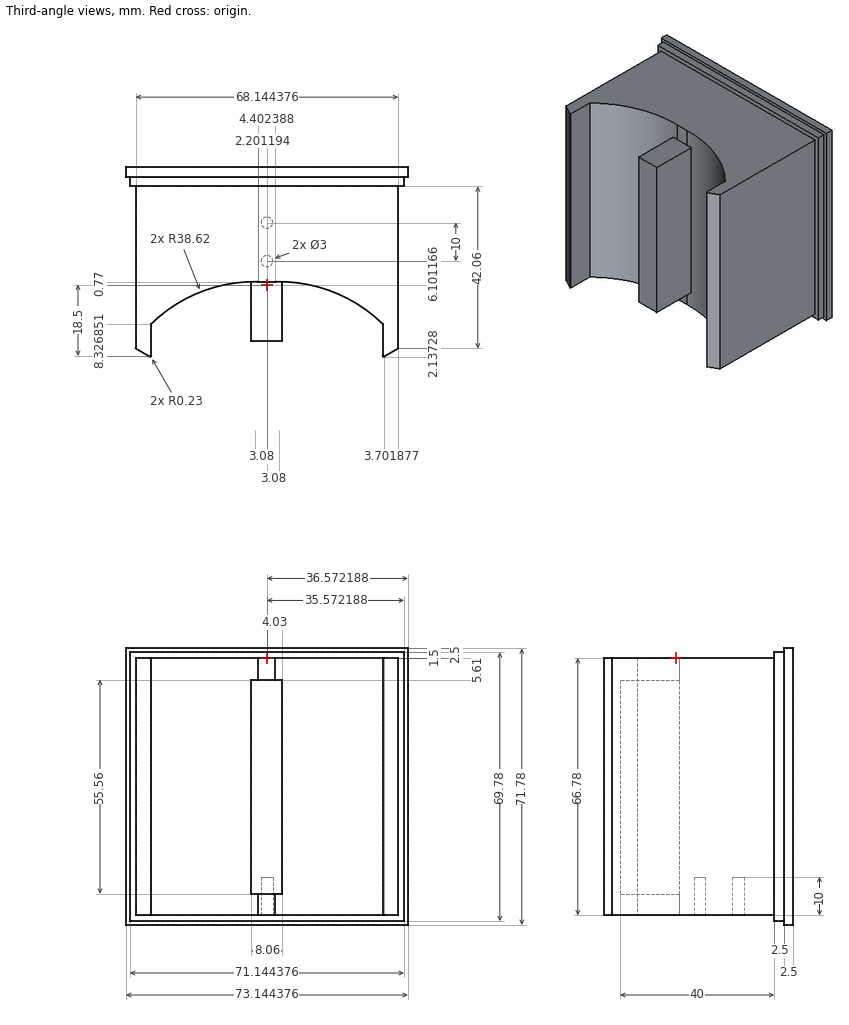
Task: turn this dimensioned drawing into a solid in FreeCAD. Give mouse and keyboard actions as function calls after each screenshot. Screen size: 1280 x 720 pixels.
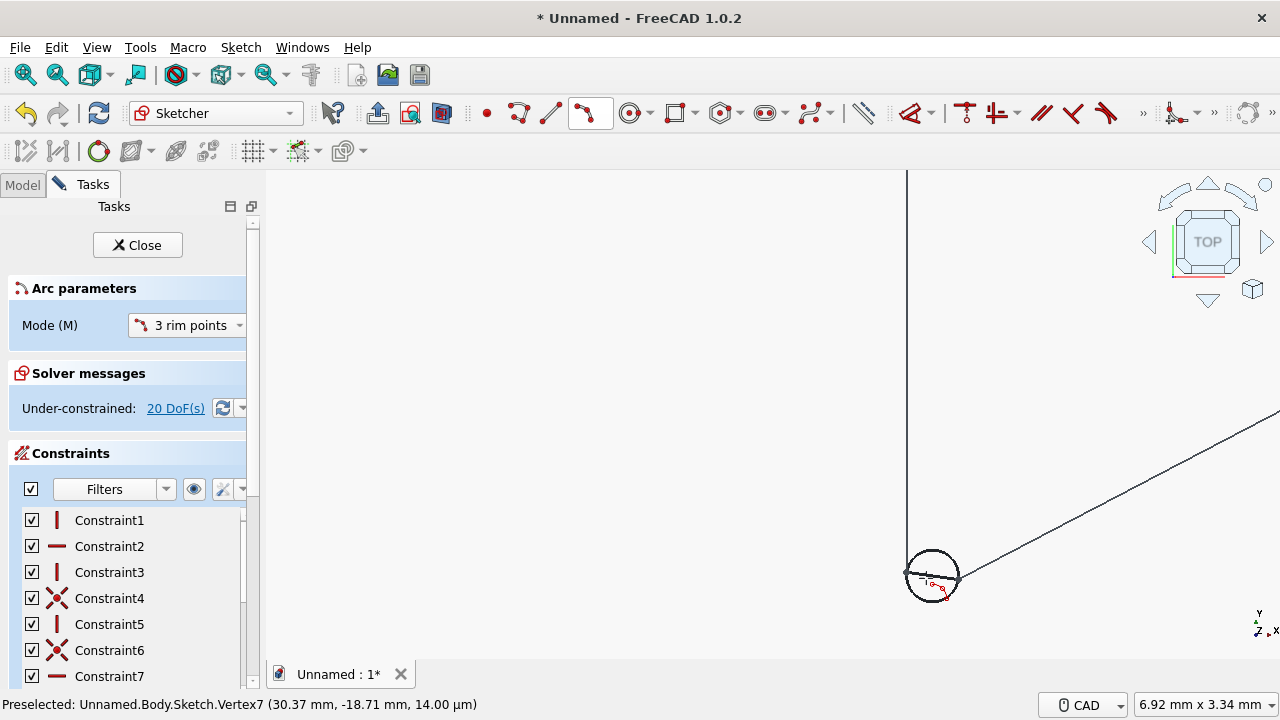
click(925, 577)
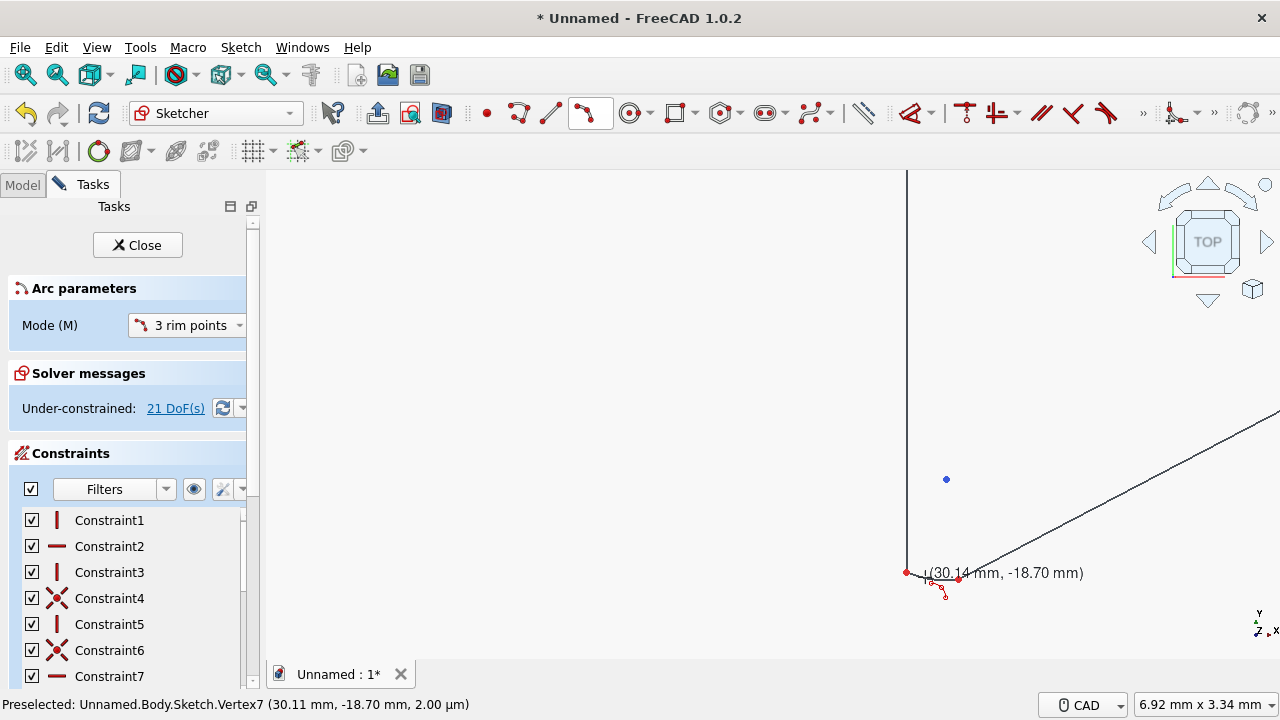
scroll(924, 576, down, 15)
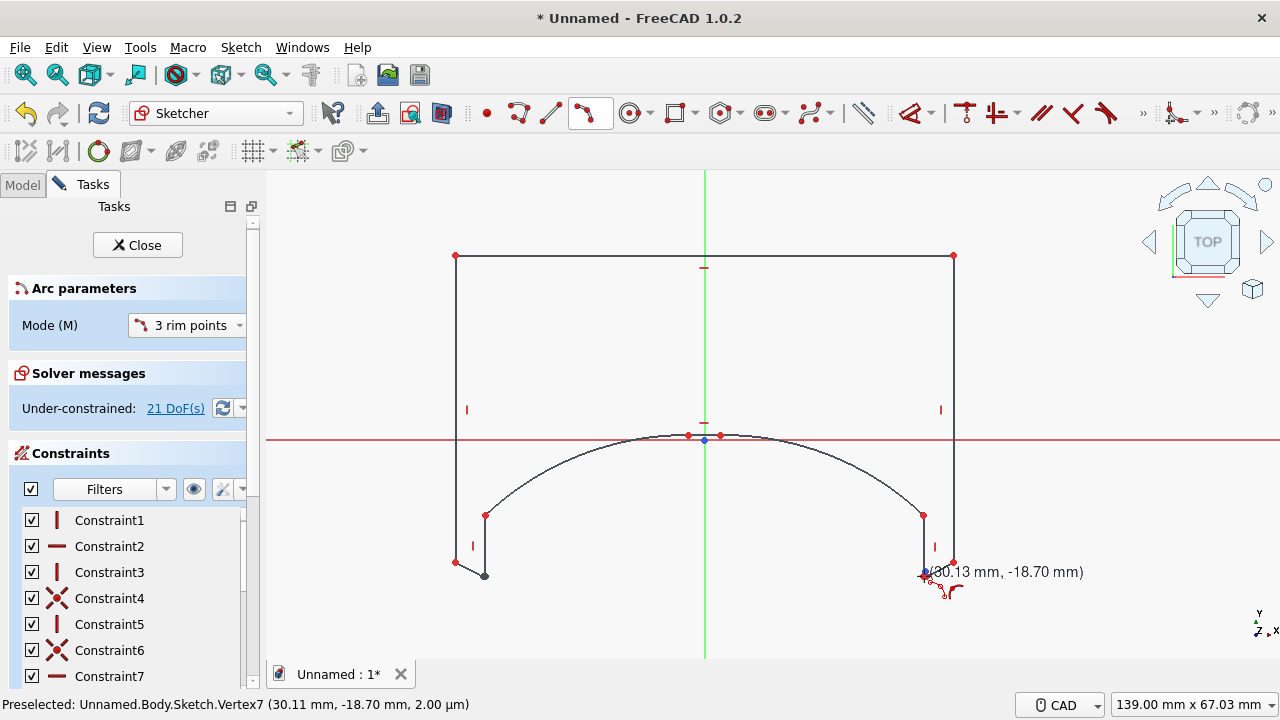
scroll(483, 577, up, 9)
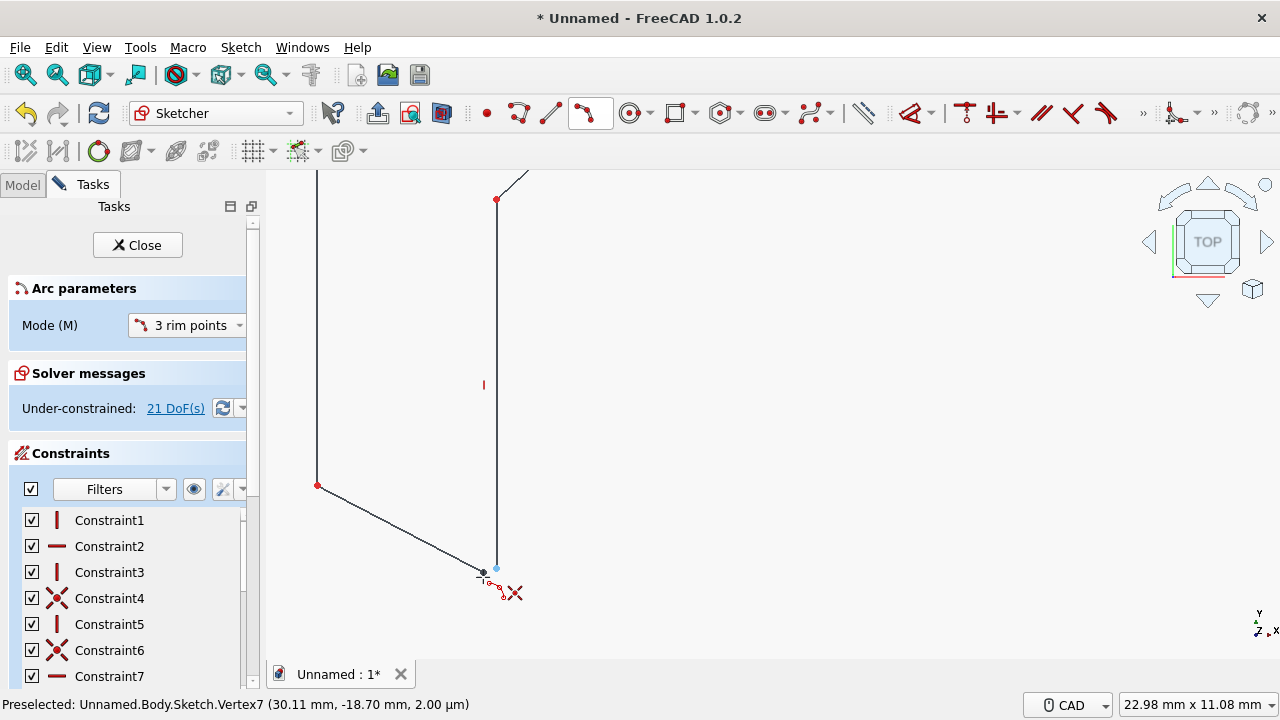
click(484, 573)
click(497, 569)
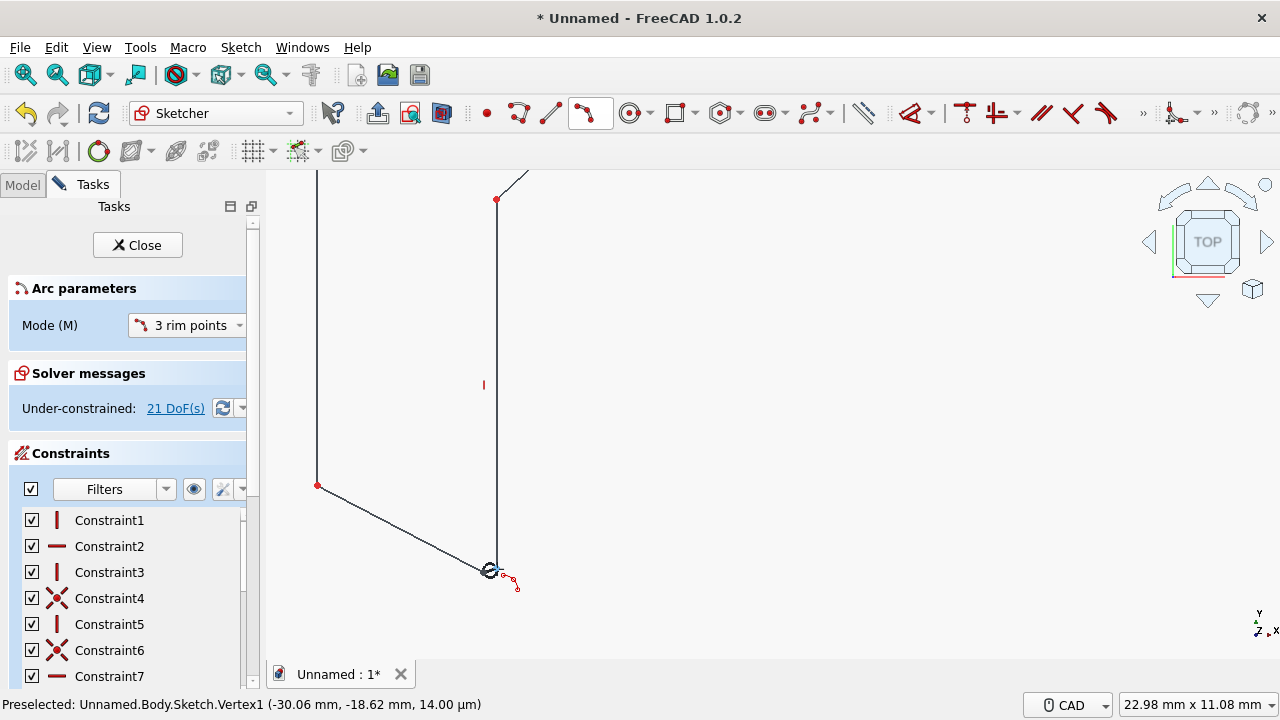
scroll(494, 572, up, 6)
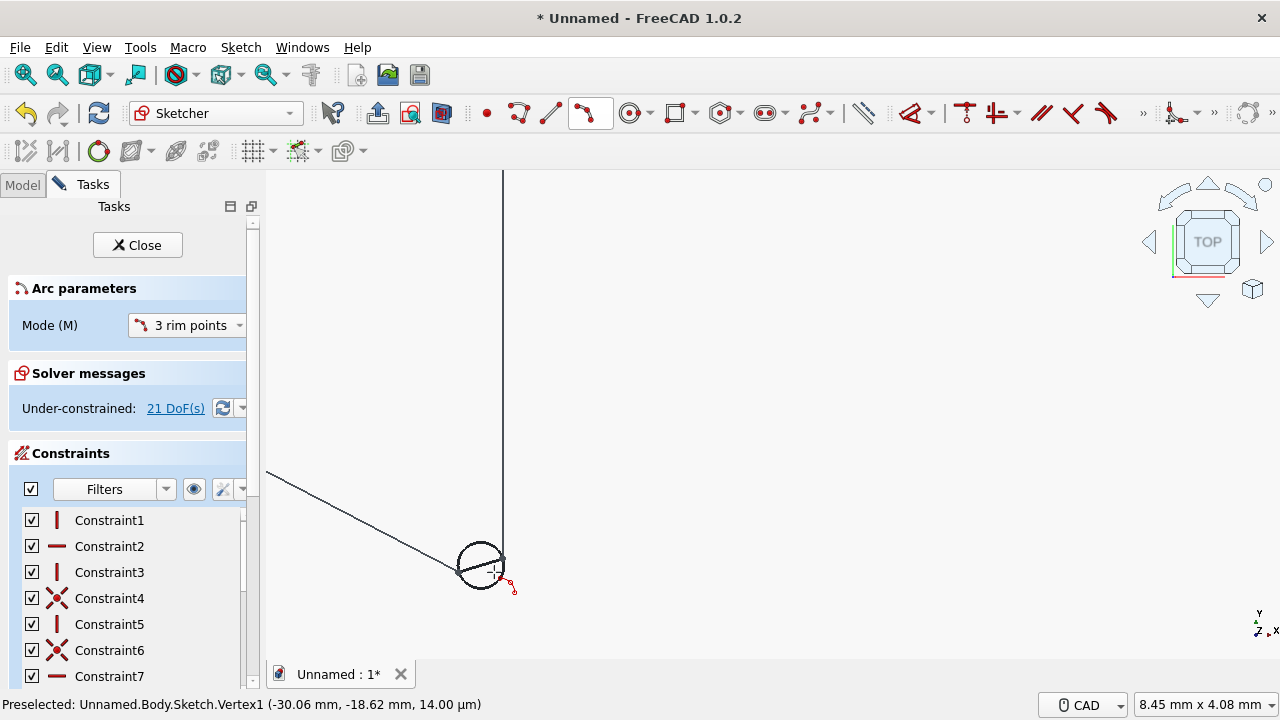
click(492, 570)
key(Escape)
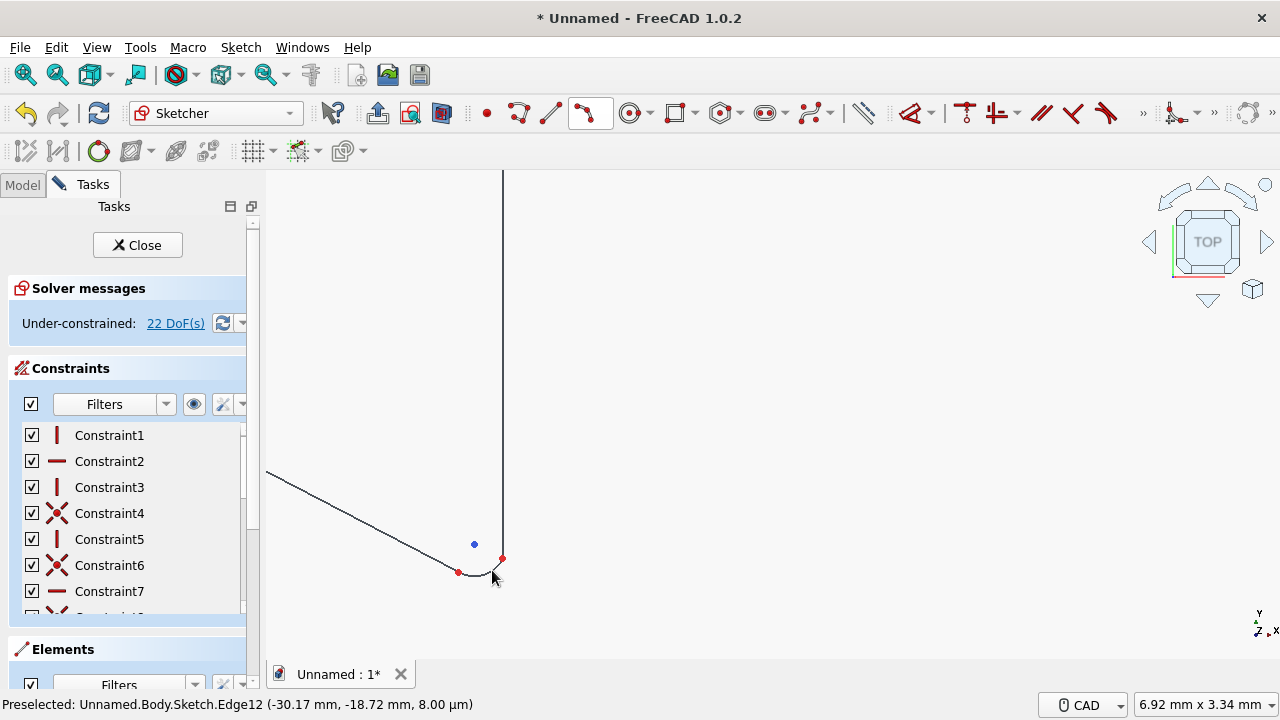
scroll(484, 576, down, 15)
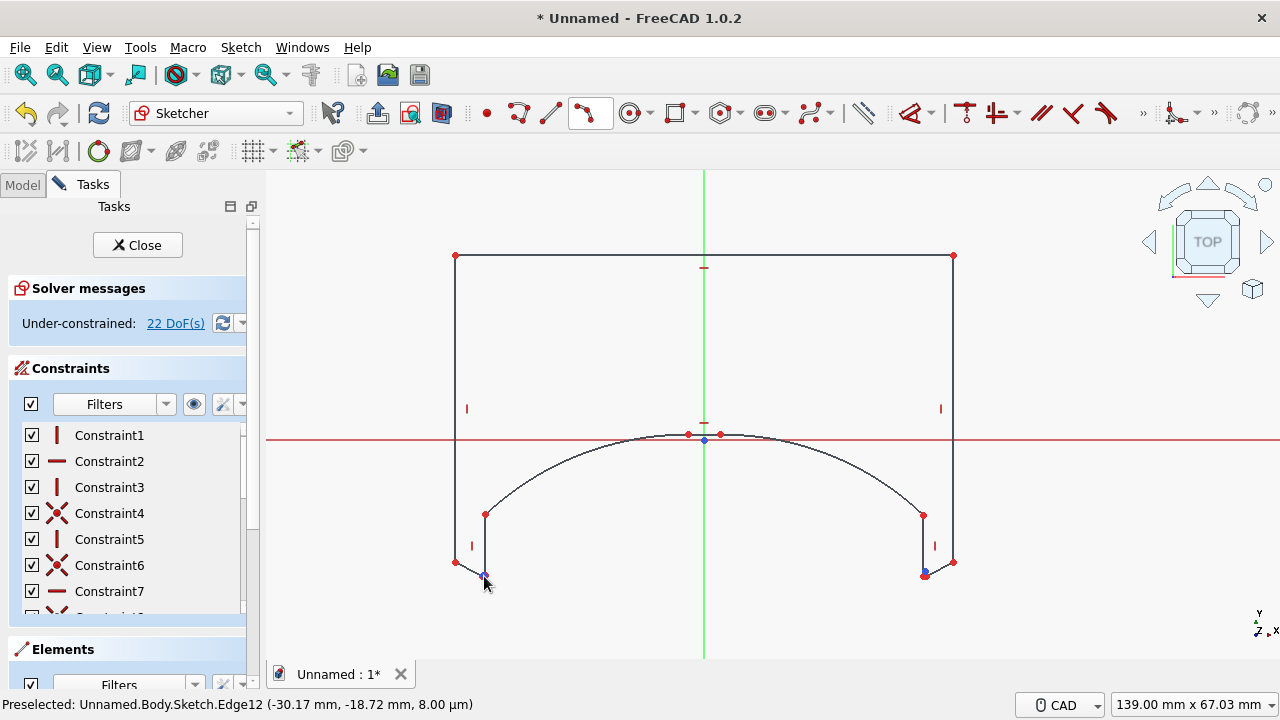
click(485, 564)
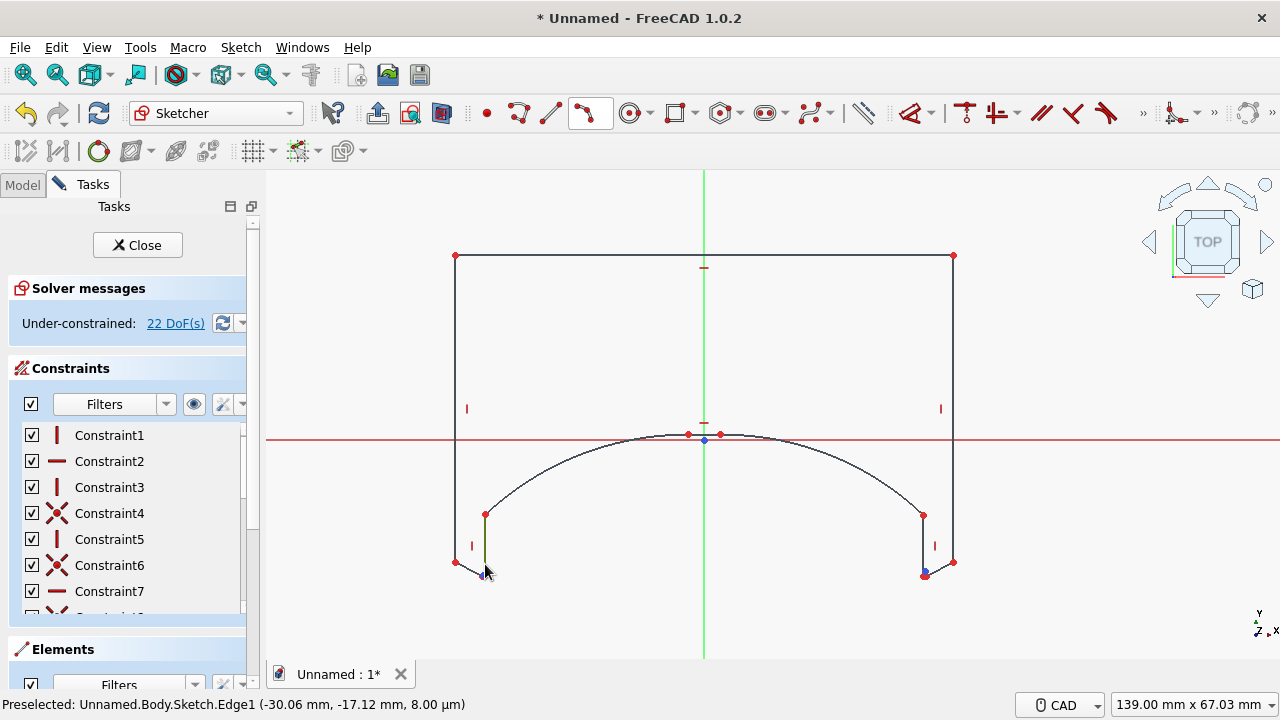
scroll(484, 577, up, 13)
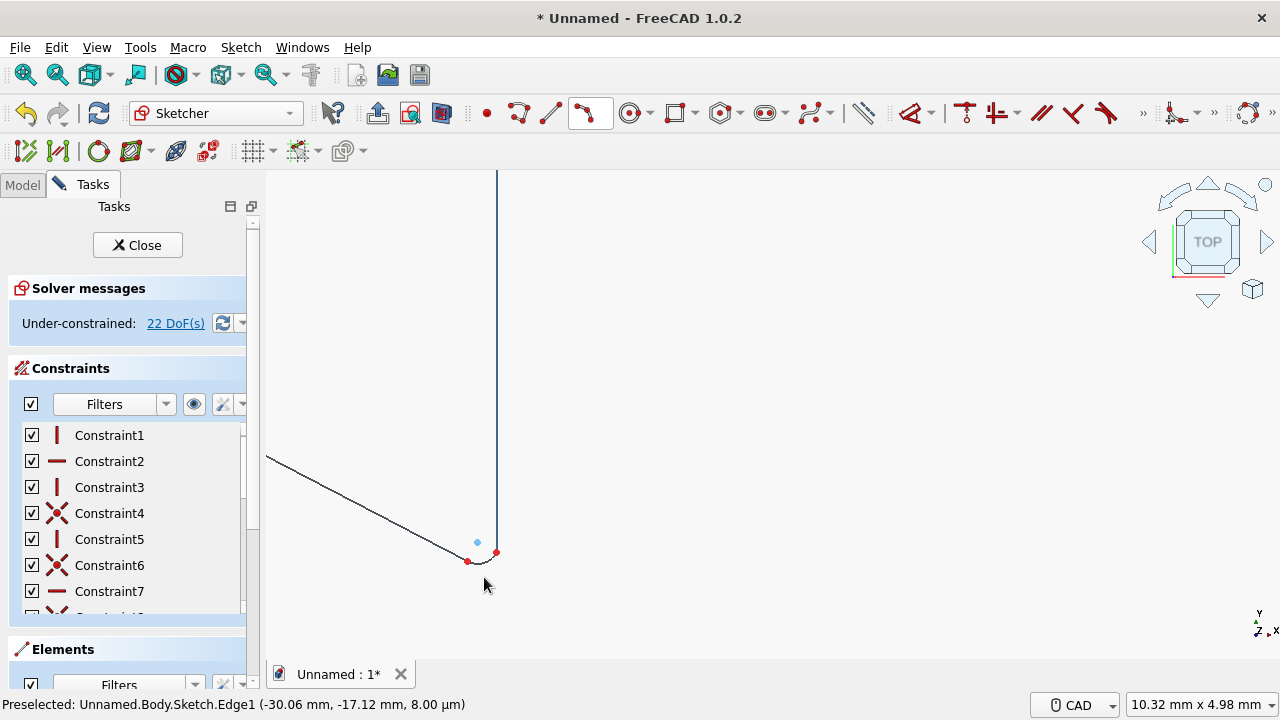
click(484, 563)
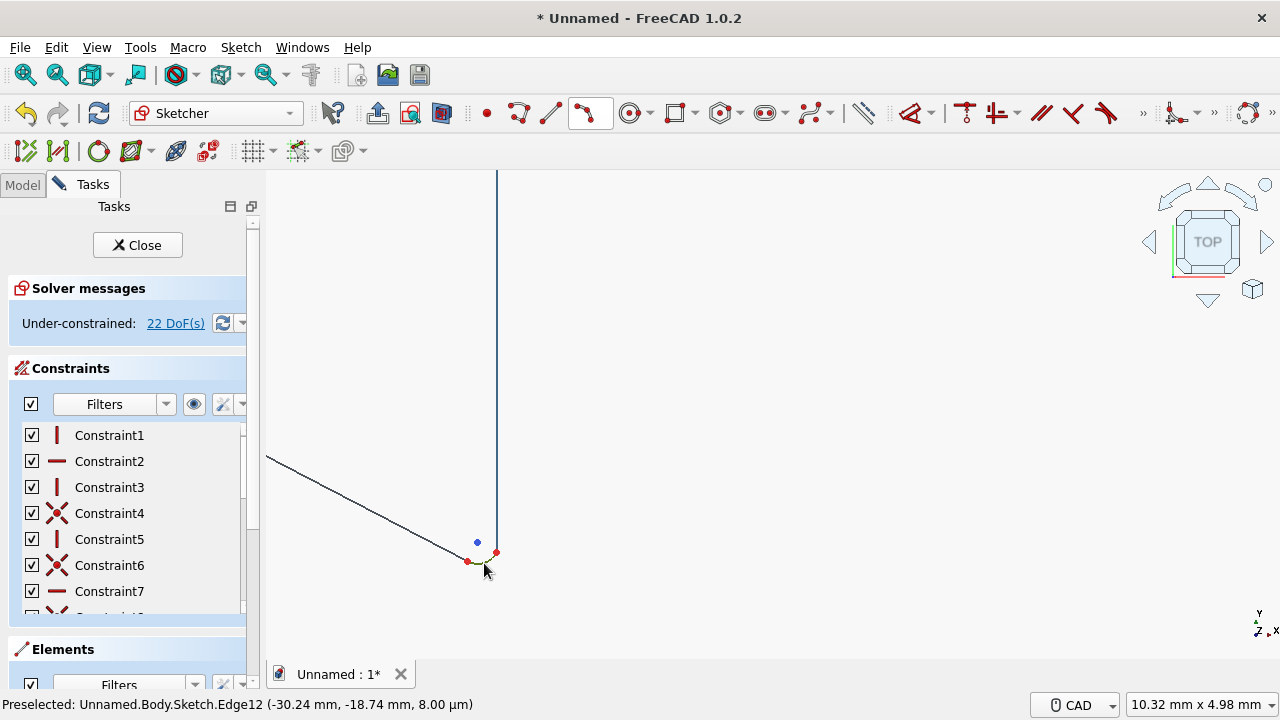
click(1106, 114)